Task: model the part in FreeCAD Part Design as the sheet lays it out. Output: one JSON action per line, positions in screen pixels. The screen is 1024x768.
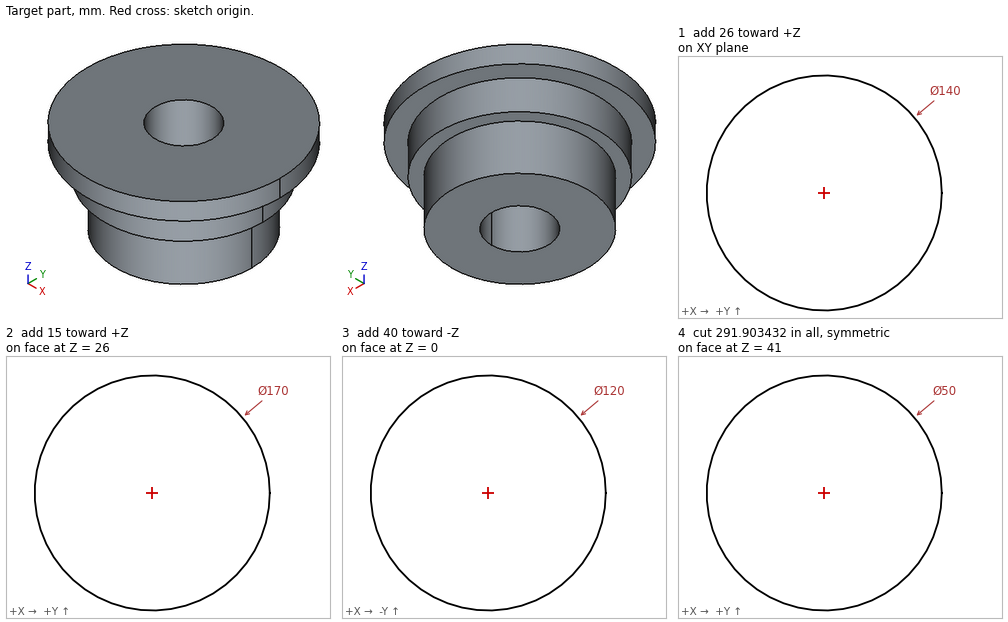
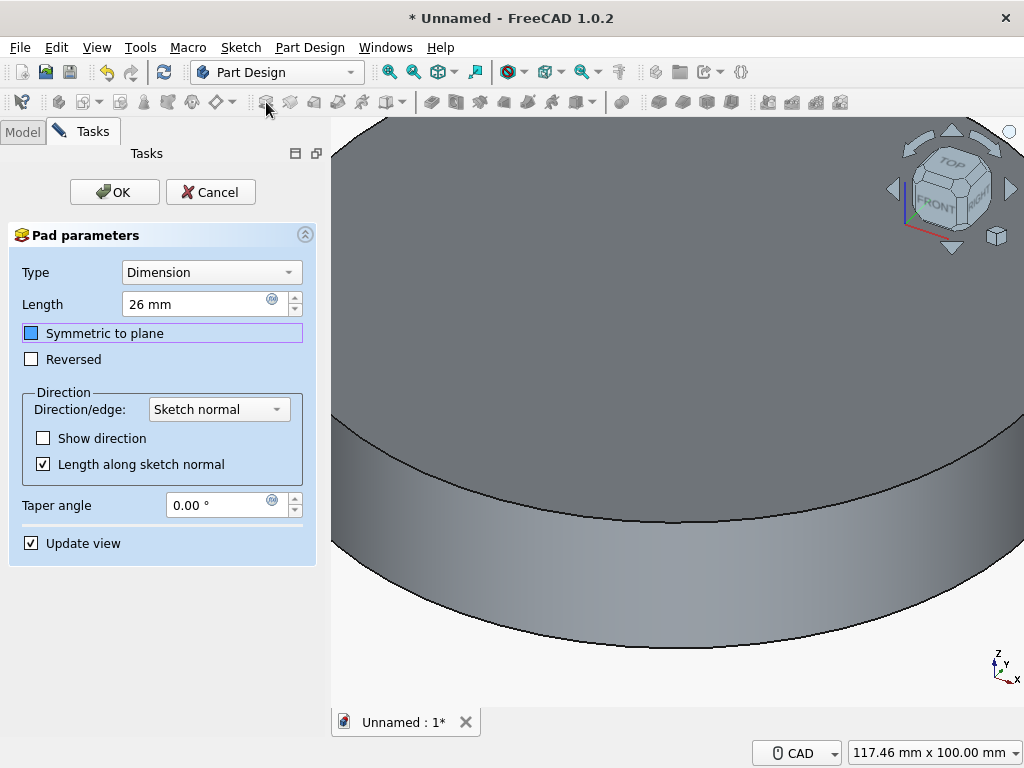
{"action": "left_click", "coordinate": [115, 192]}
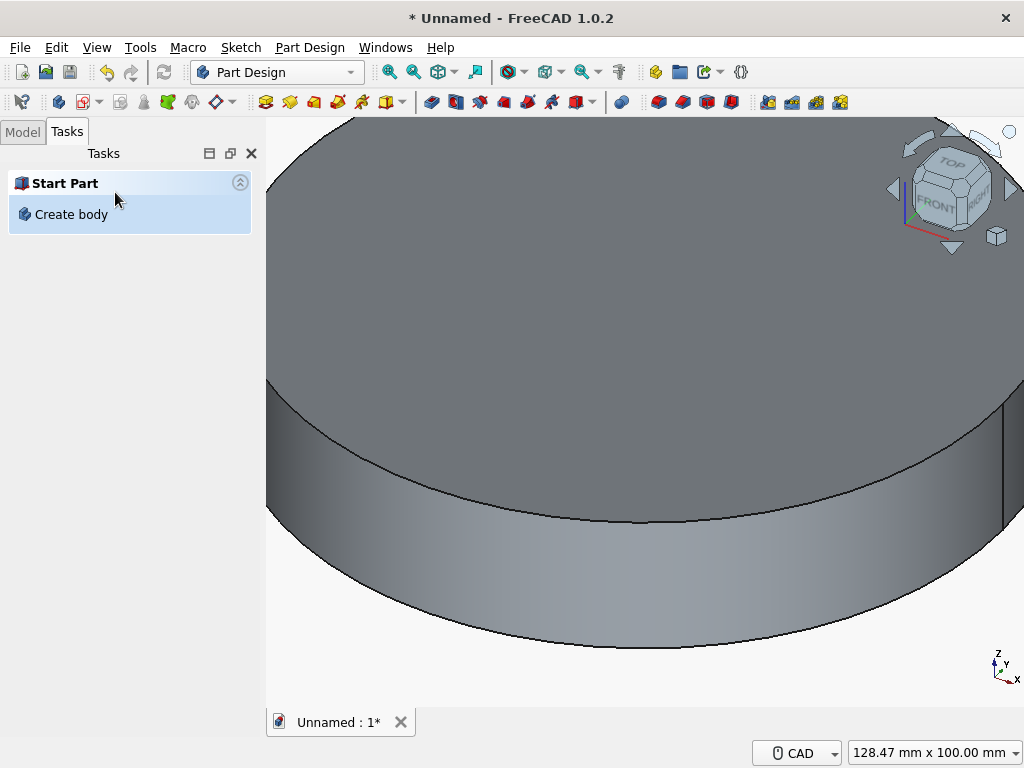
{"action": "key", "text": "v f"}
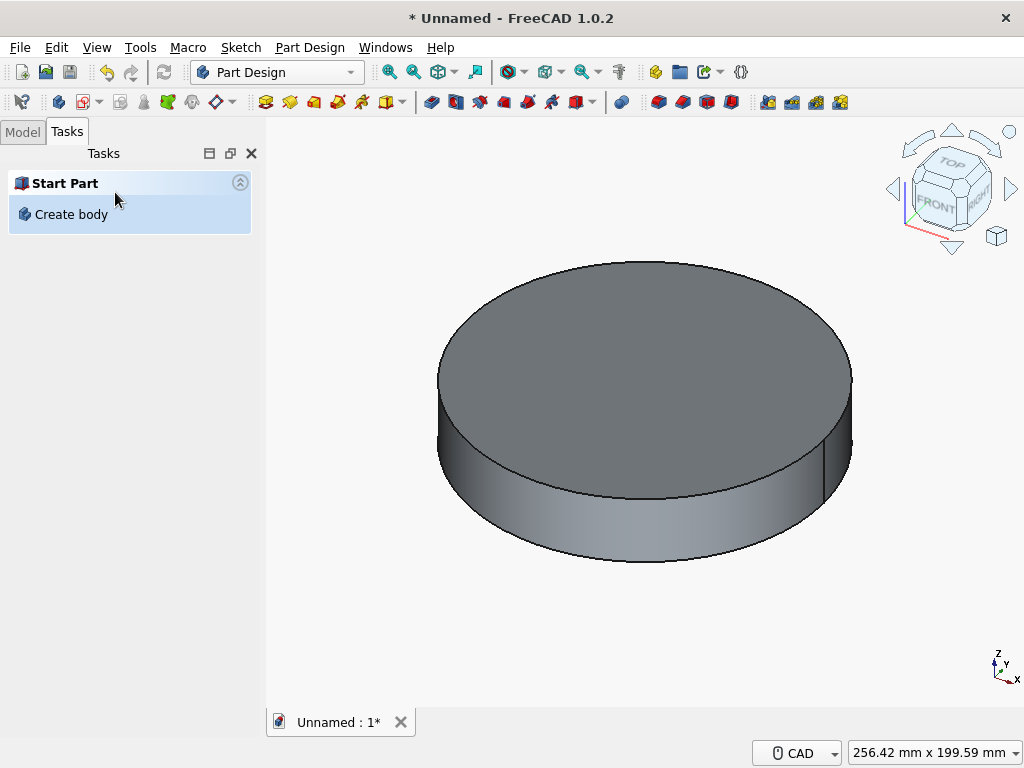
{"action": "left_click", "coordinate": [645, 379]}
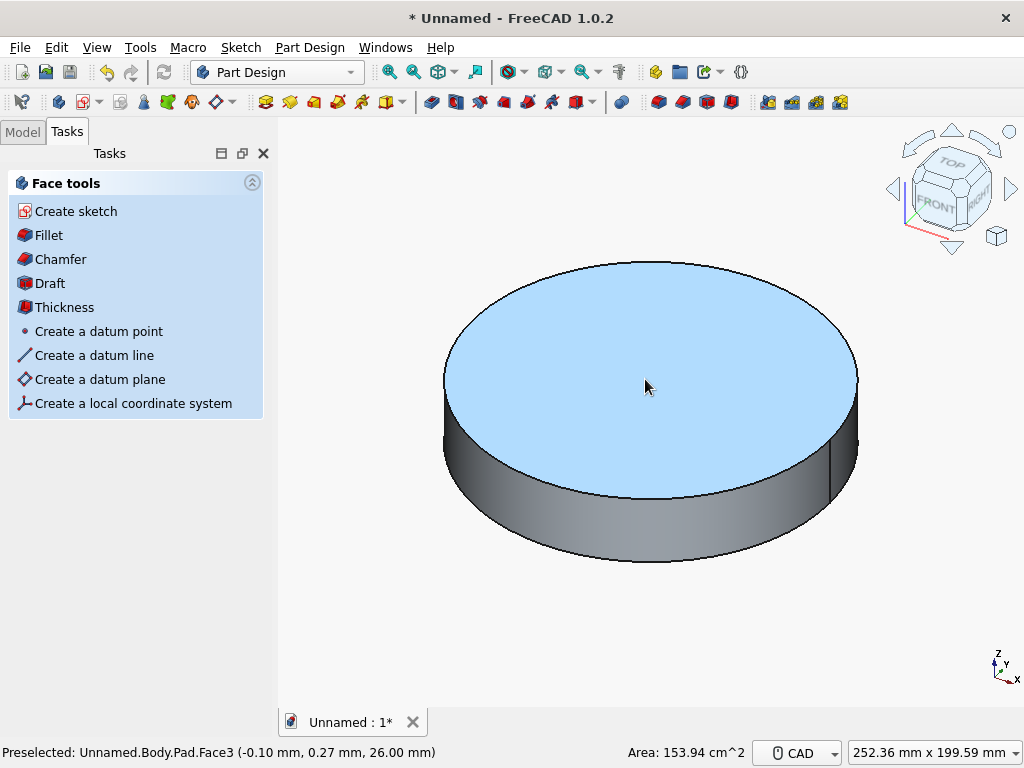
{"action": "left_click", "coordinate": [84, 102]}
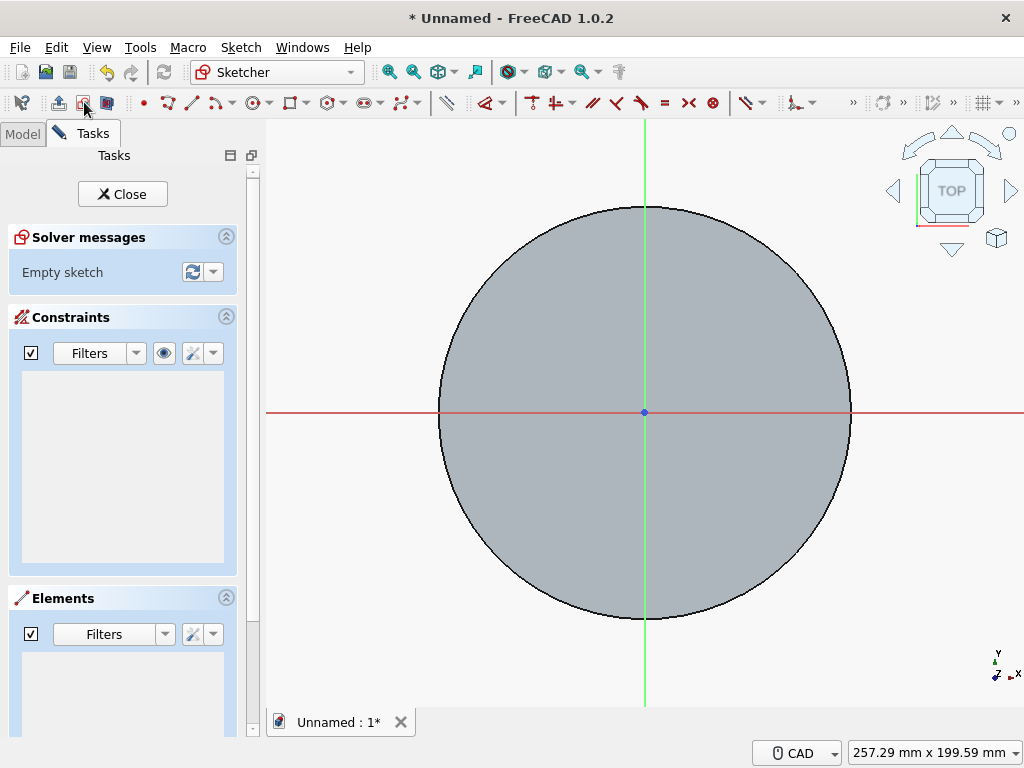
{"action": "scroll", "coordinate": [294, 413], "scroll_direction": "down", "scroll_amount": 1}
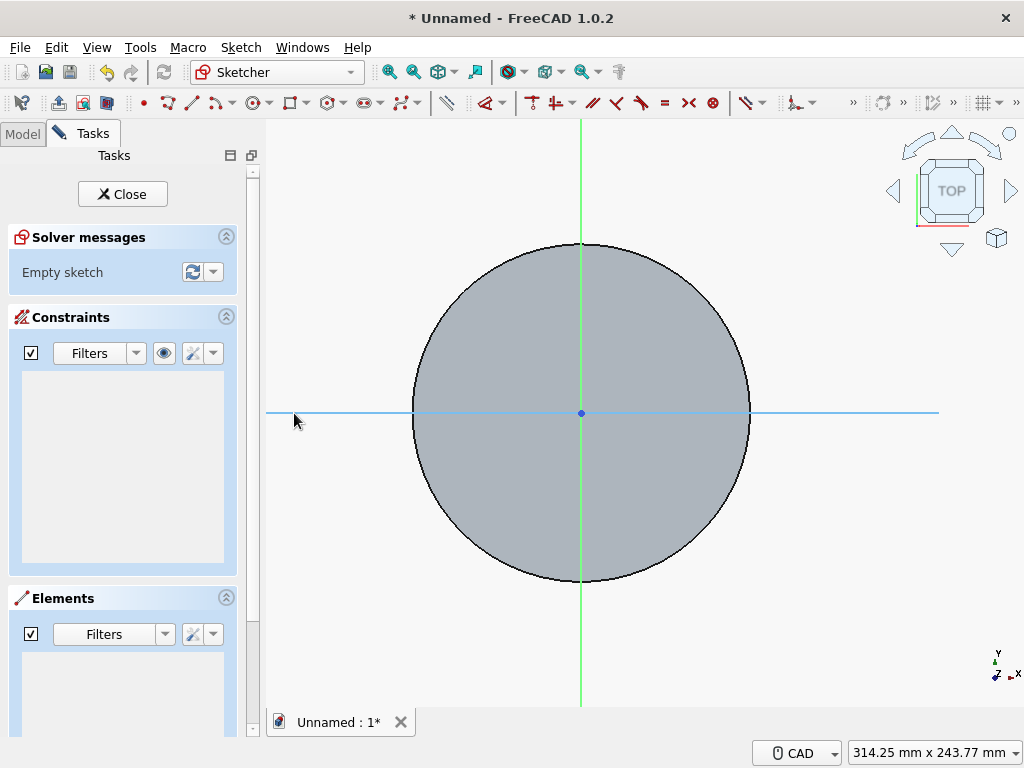
{"action": "key", "text": "g c"}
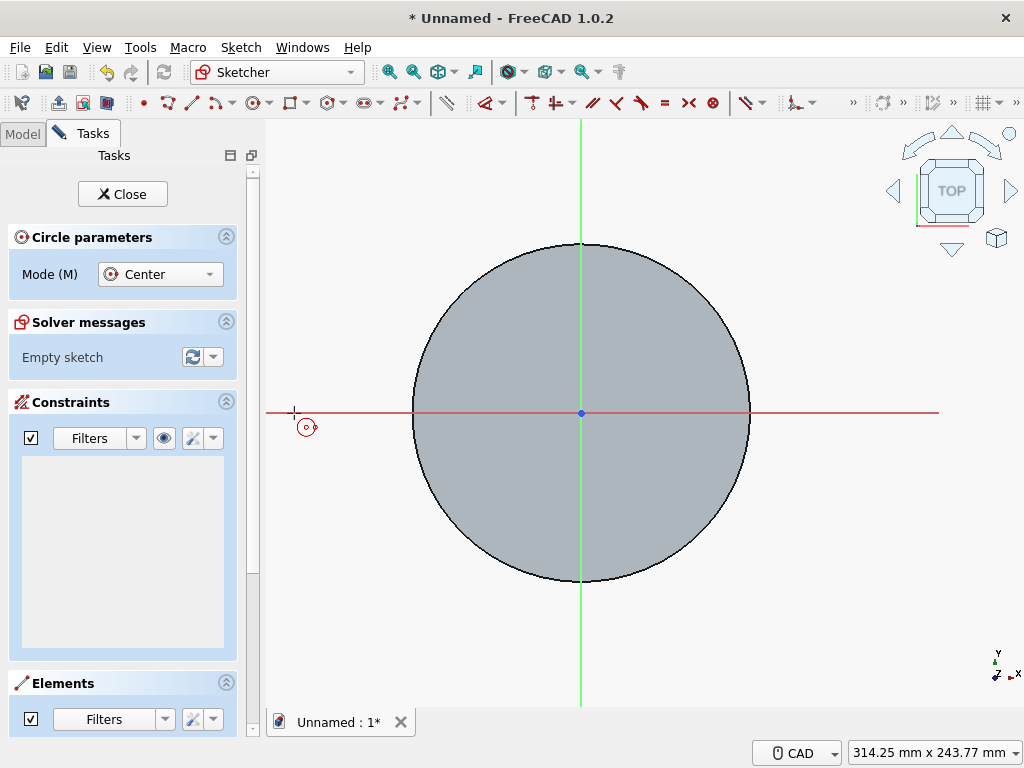
{"action": "left_click", "coordinate": [581, 413]}
{"action": "left_click", "coordinate": [726, 268]}
{"action": "key", "text": "Escape"}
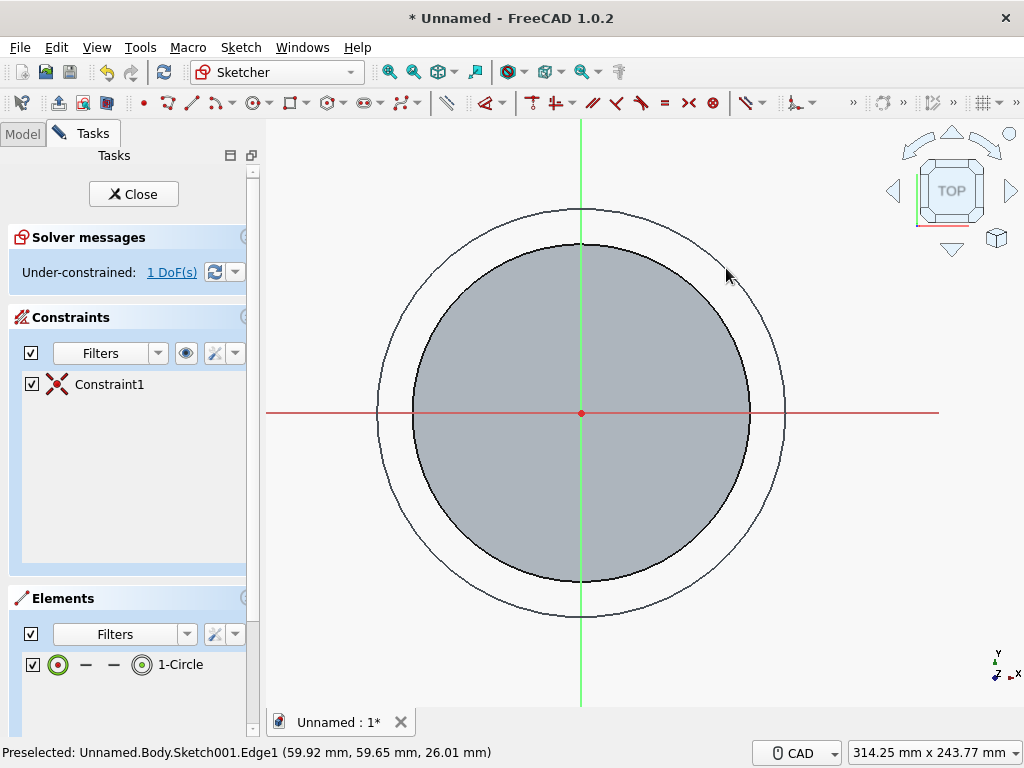
{"action": "key", "text": "d"}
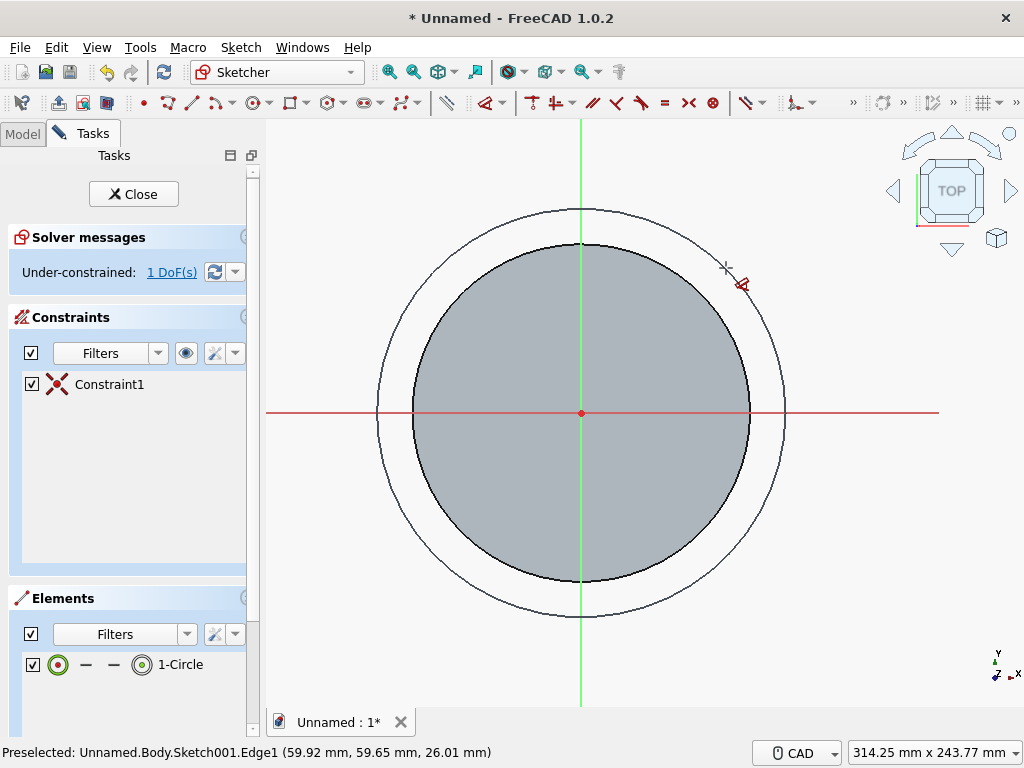
{"action": "left_click", "coordinate": [725, 268]}
{"action": "left_click", "coordinate": [748, 245]}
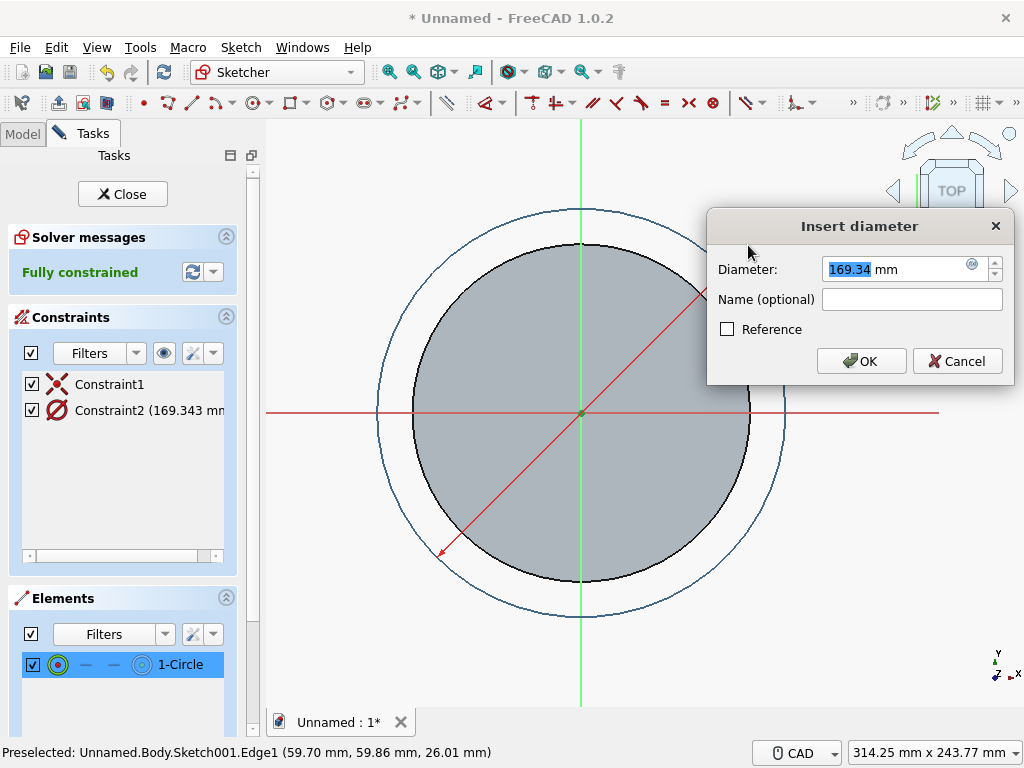
{"action": "type", "text": "170"}
{"action": "key", "text": "Return"}
{"action": "key", "text": "Escape"}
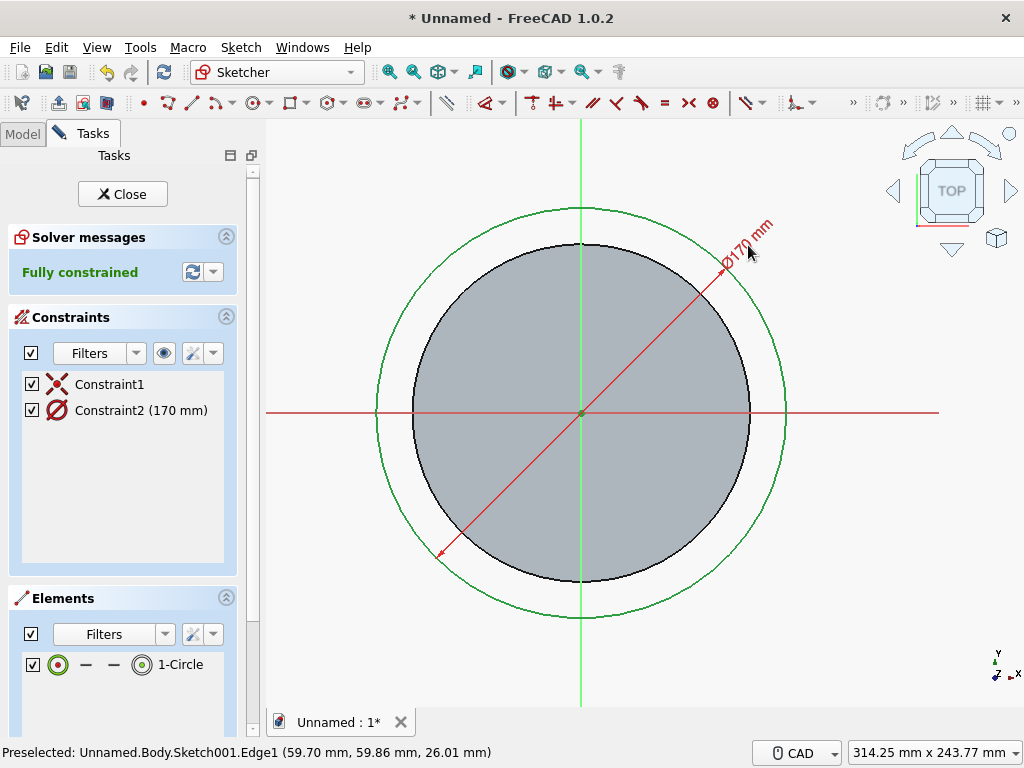
{"action": "left_click", "coordinate": [123, 194]}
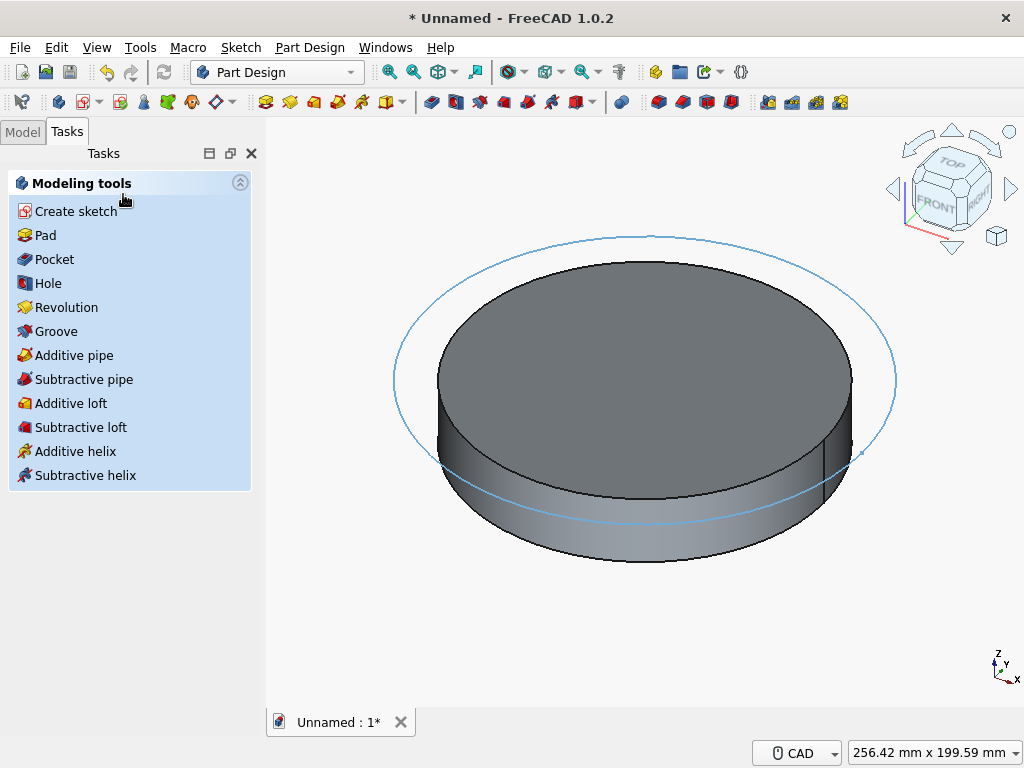
{"action": "left_click", "coordinate": [266, 102]}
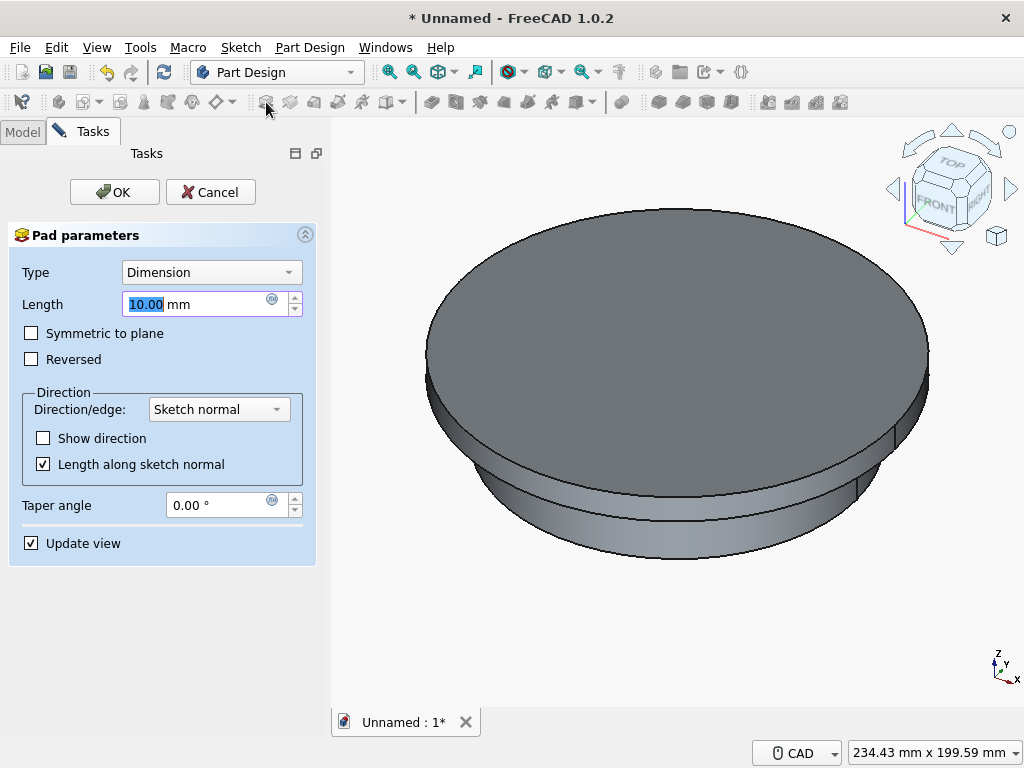
{"action": "type", "text": "15"}
{"action": "key", "text": "Tab"}